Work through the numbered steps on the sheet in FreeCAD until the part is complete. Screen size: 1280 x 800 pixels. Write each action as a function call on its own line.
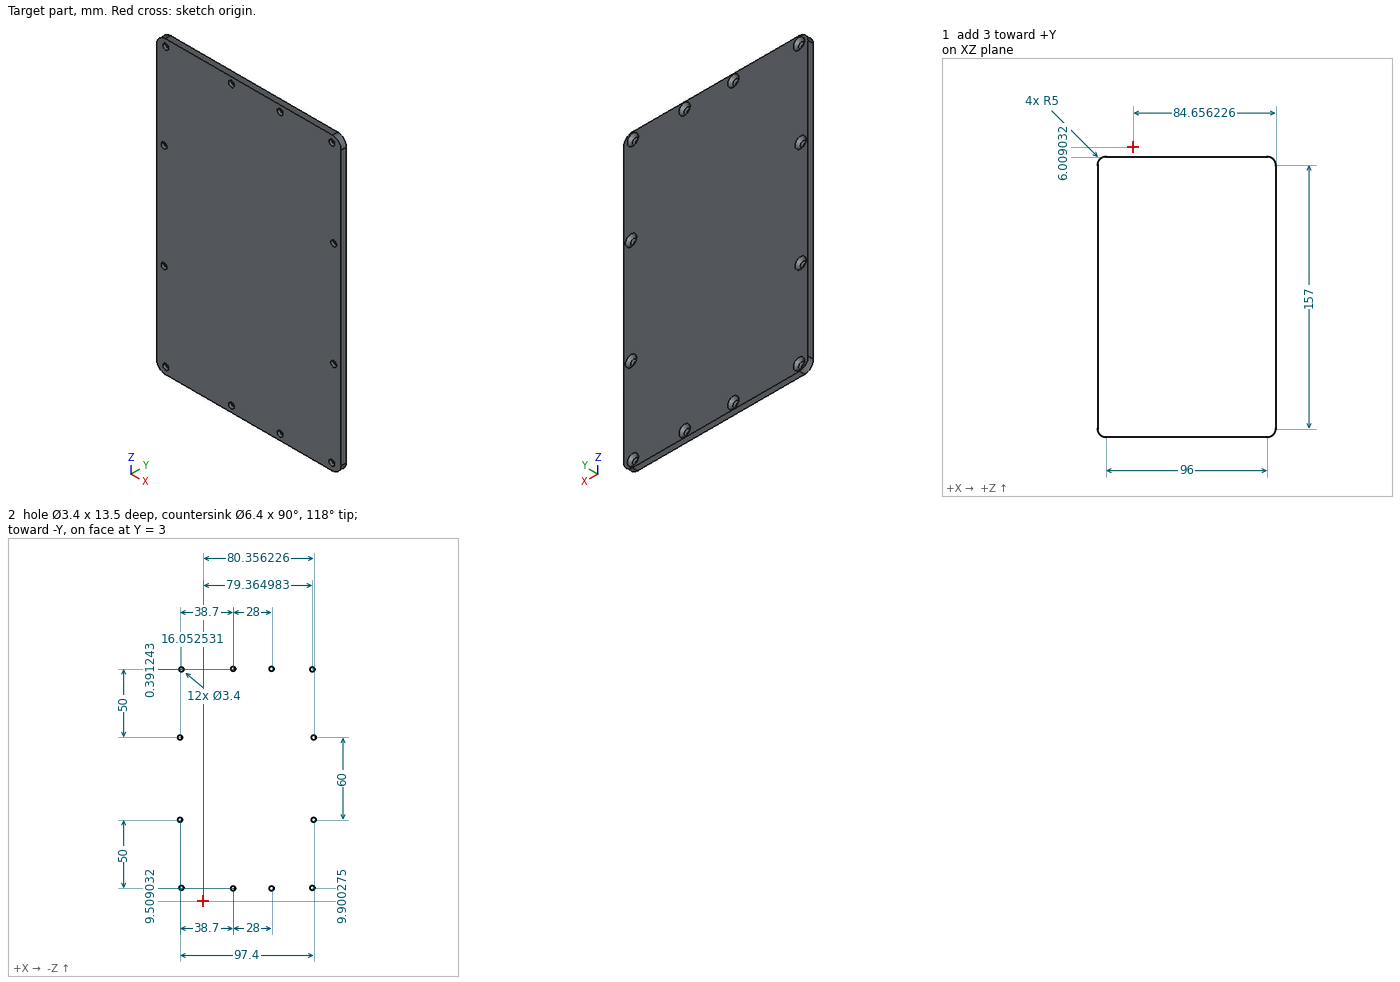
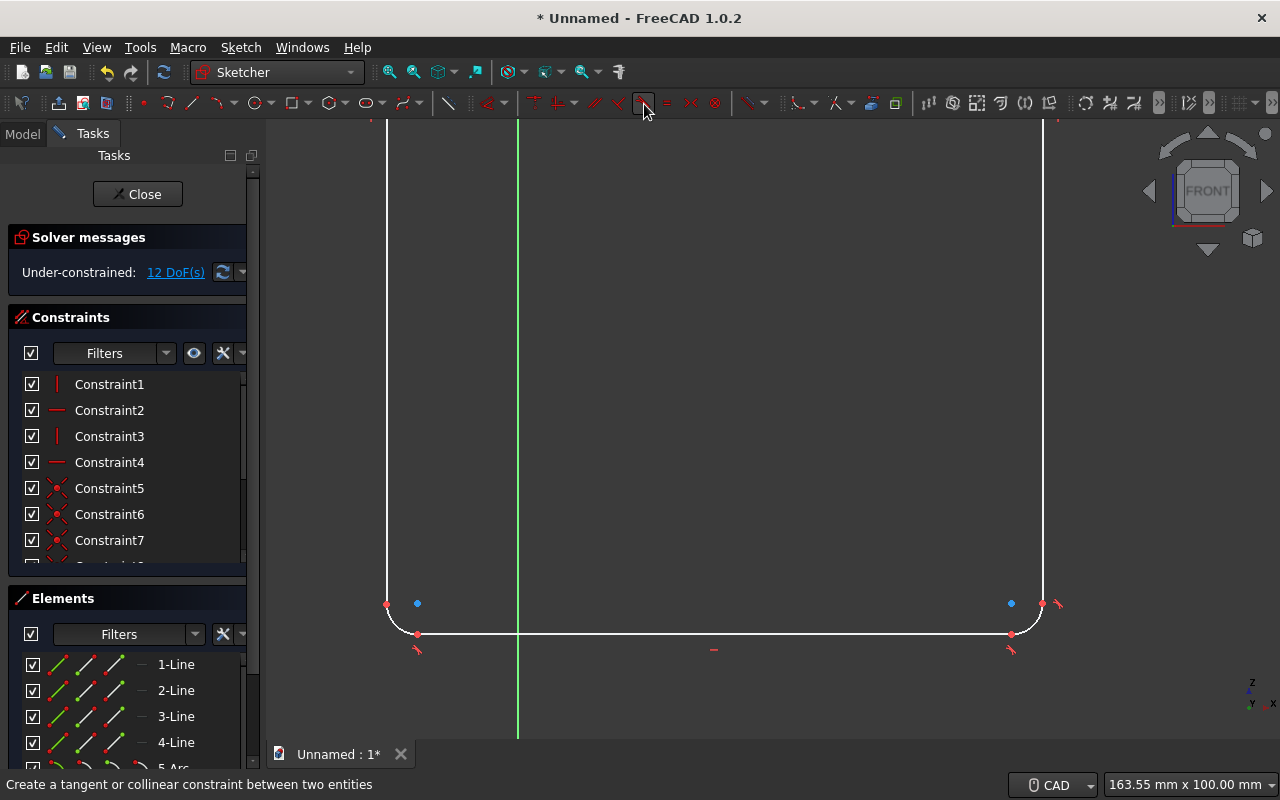
click(387, 313)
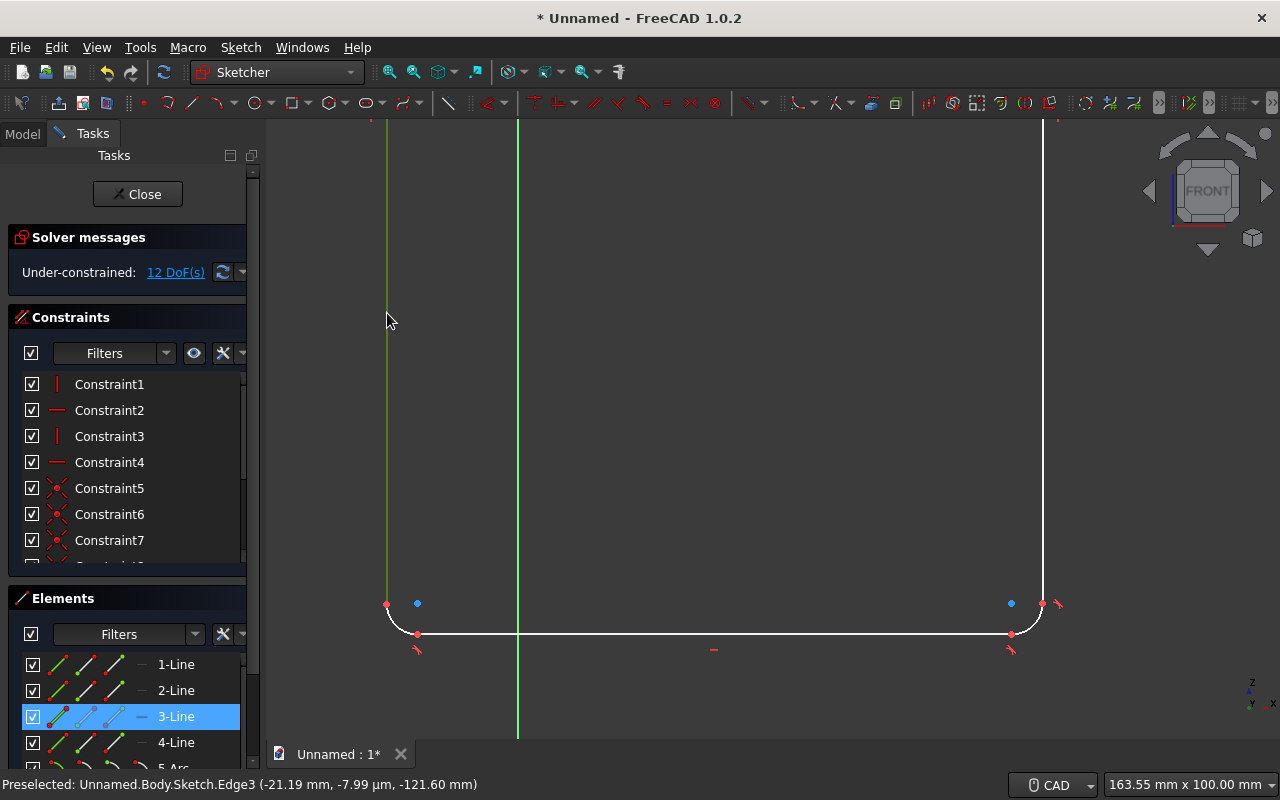
click(390, 618)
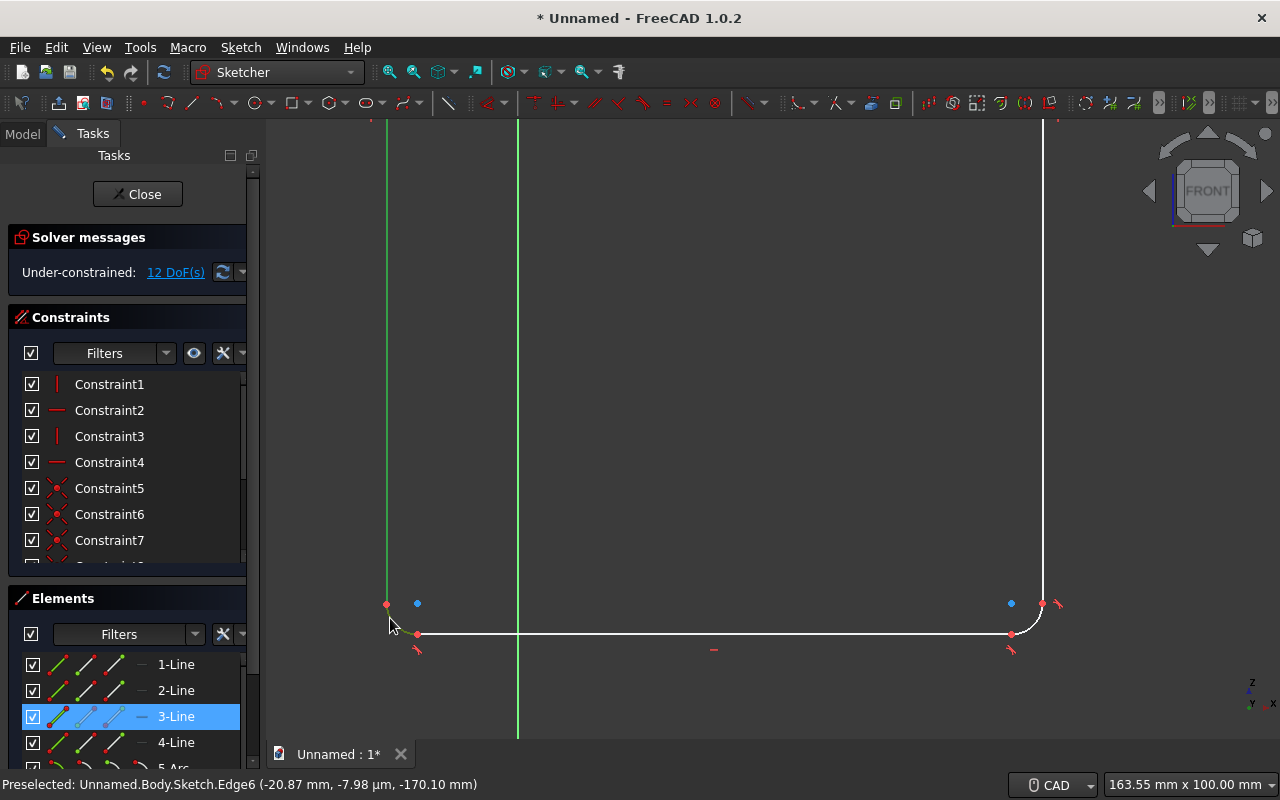
click(644, 104)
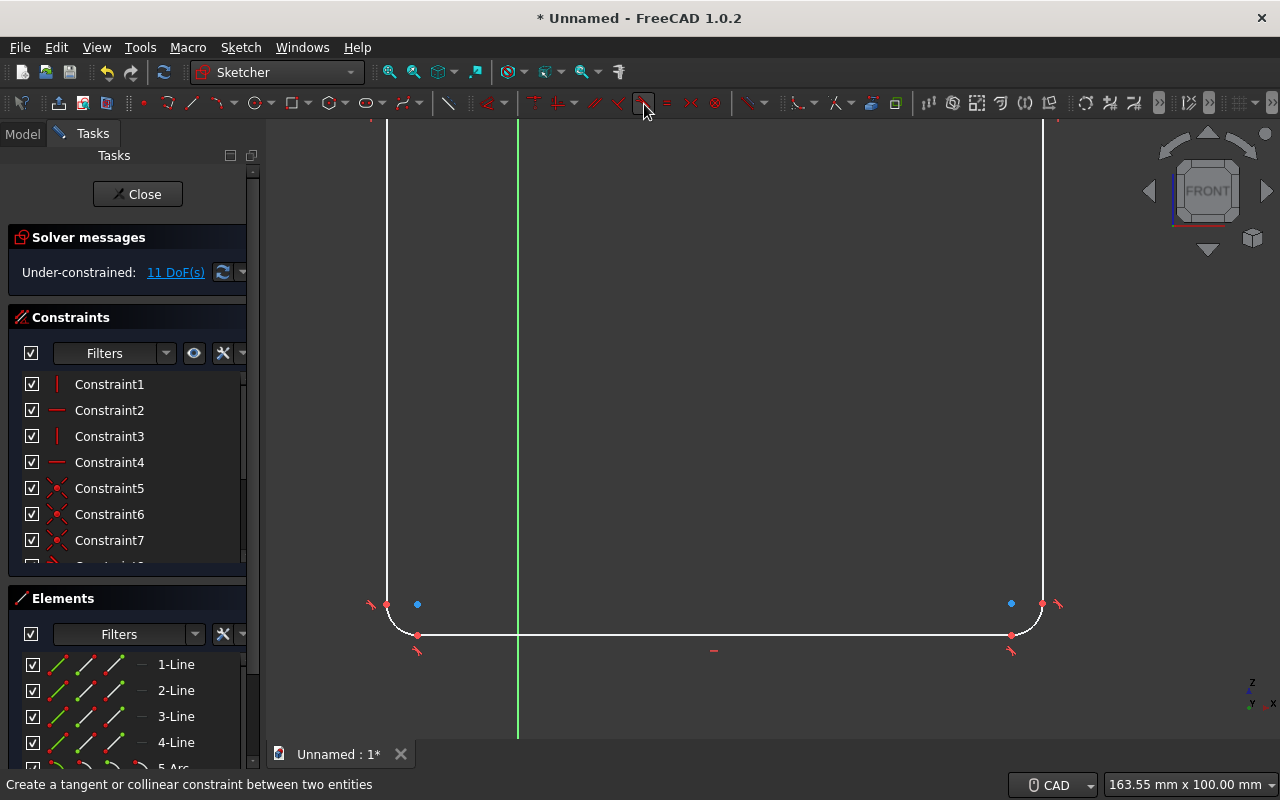
click(387, 313)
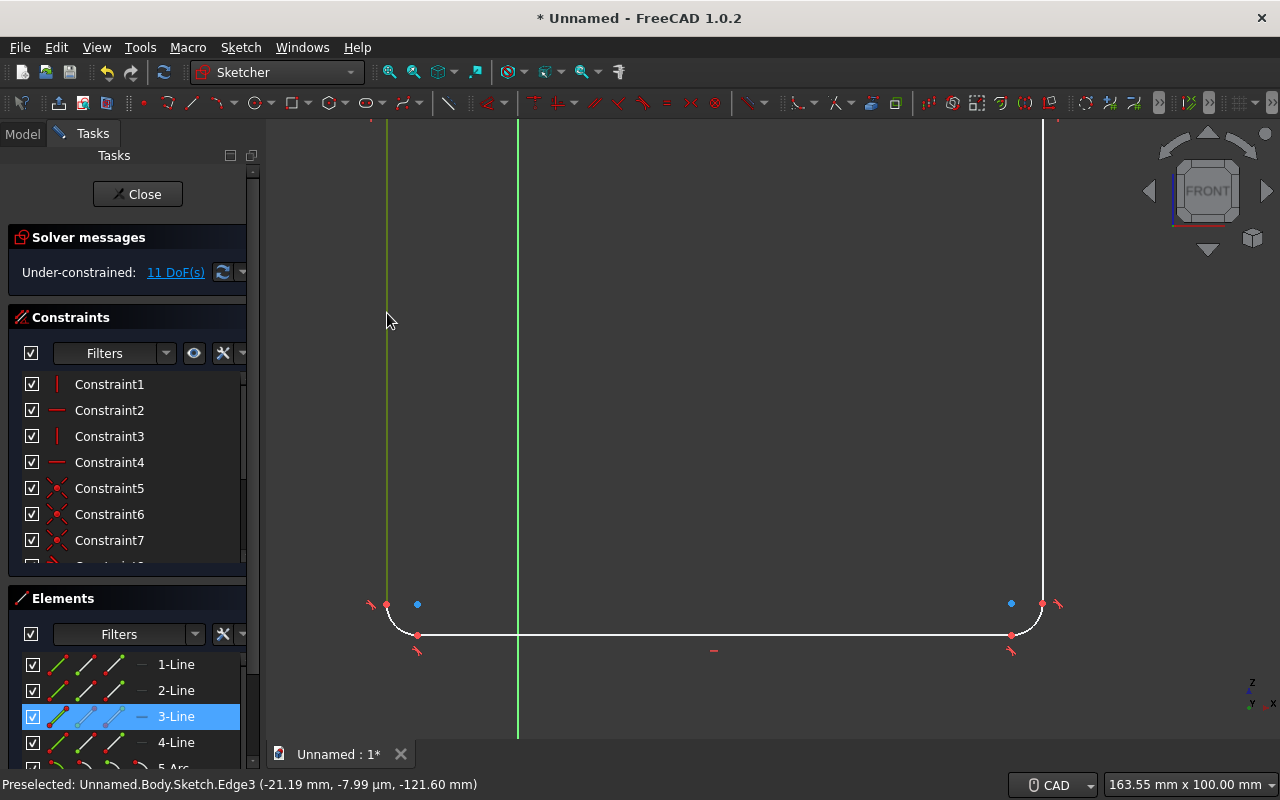
scroll(699, 623, down, 5)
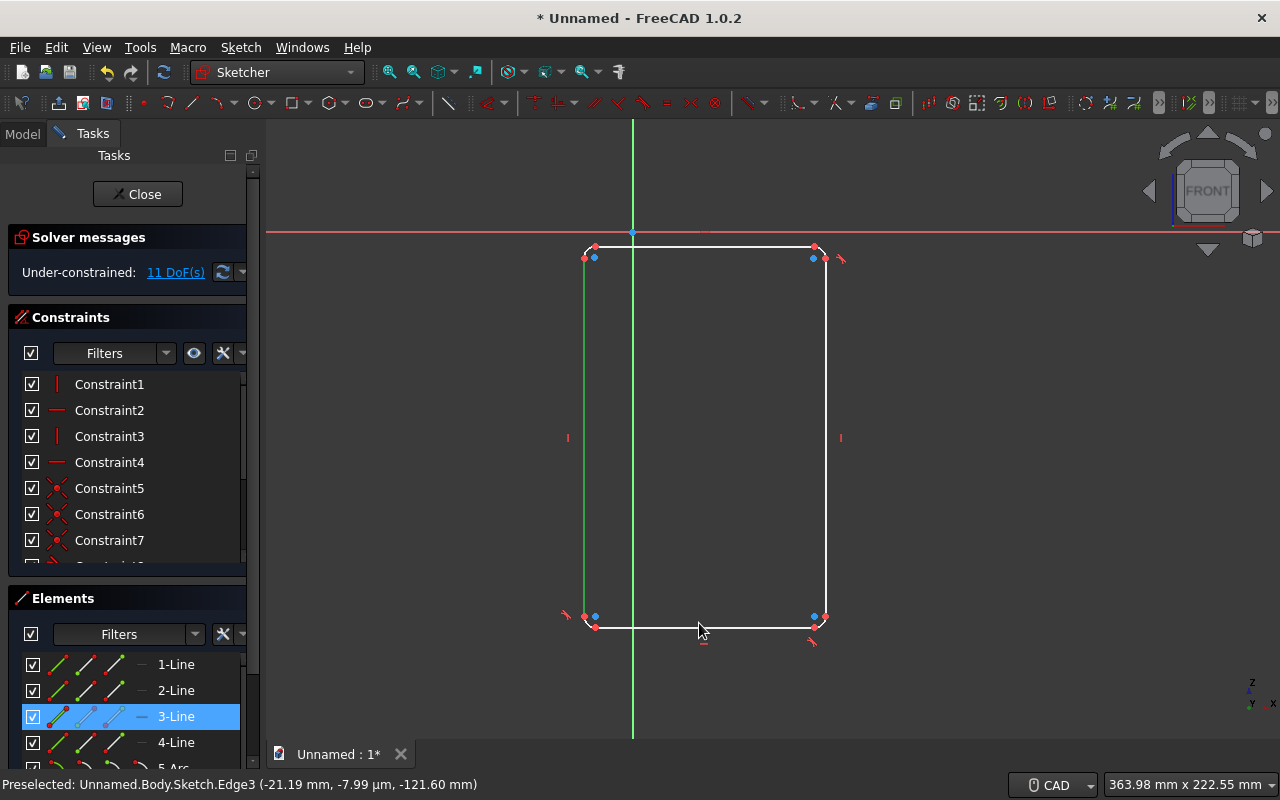
scroll(590, 248, up, 5)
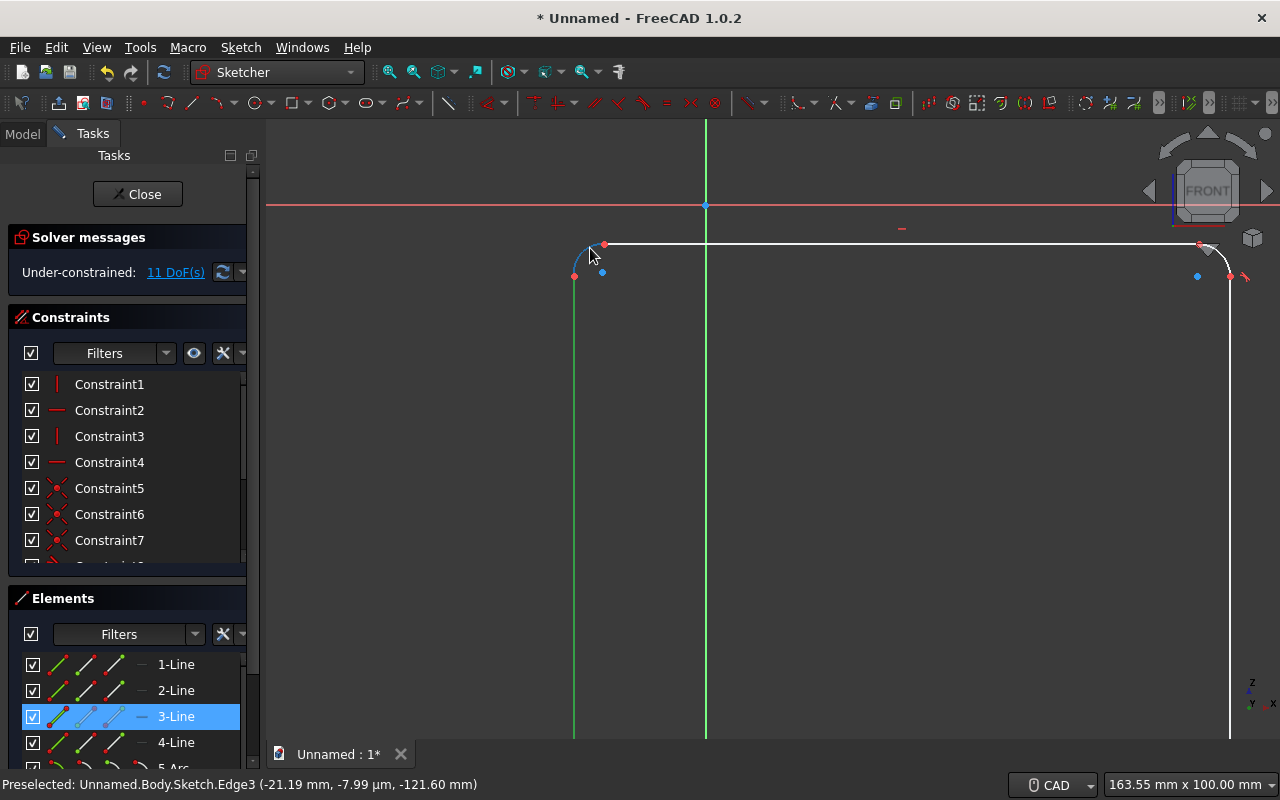
click(590, 247)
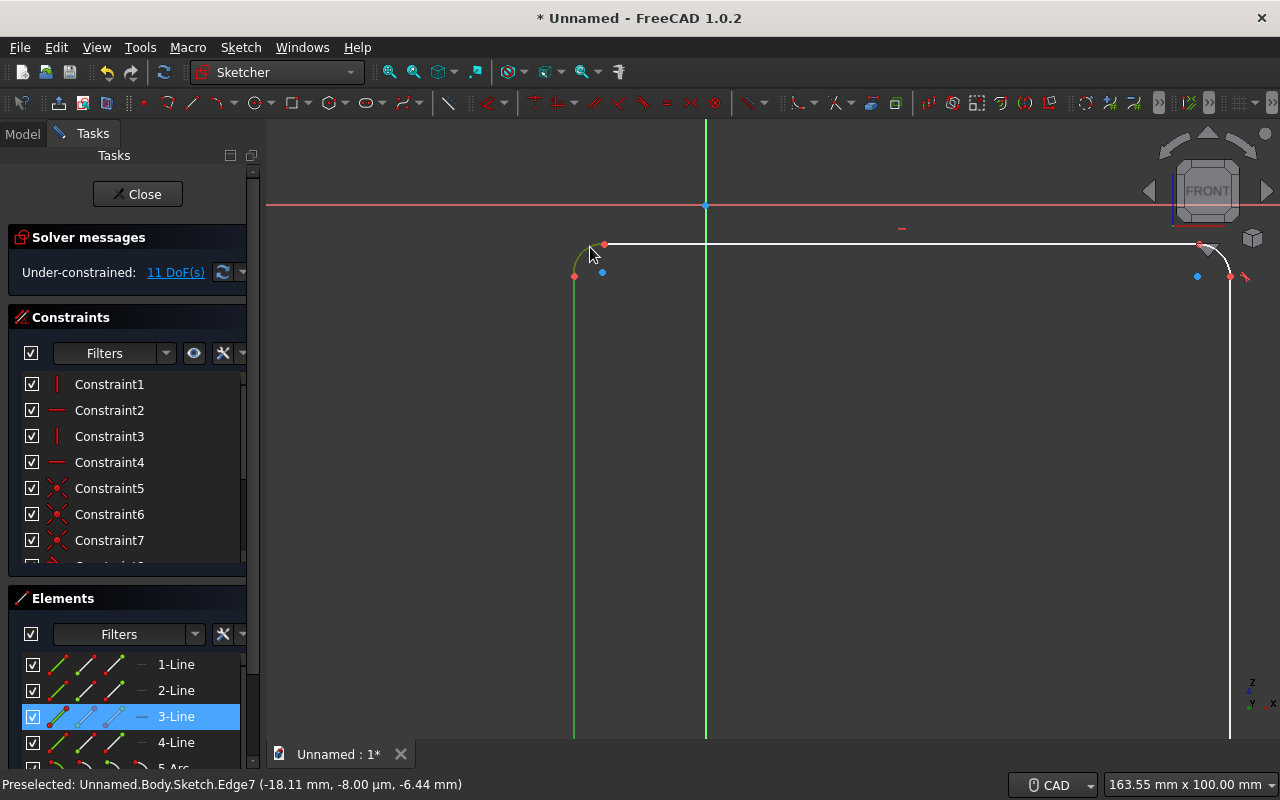
click(644, 104)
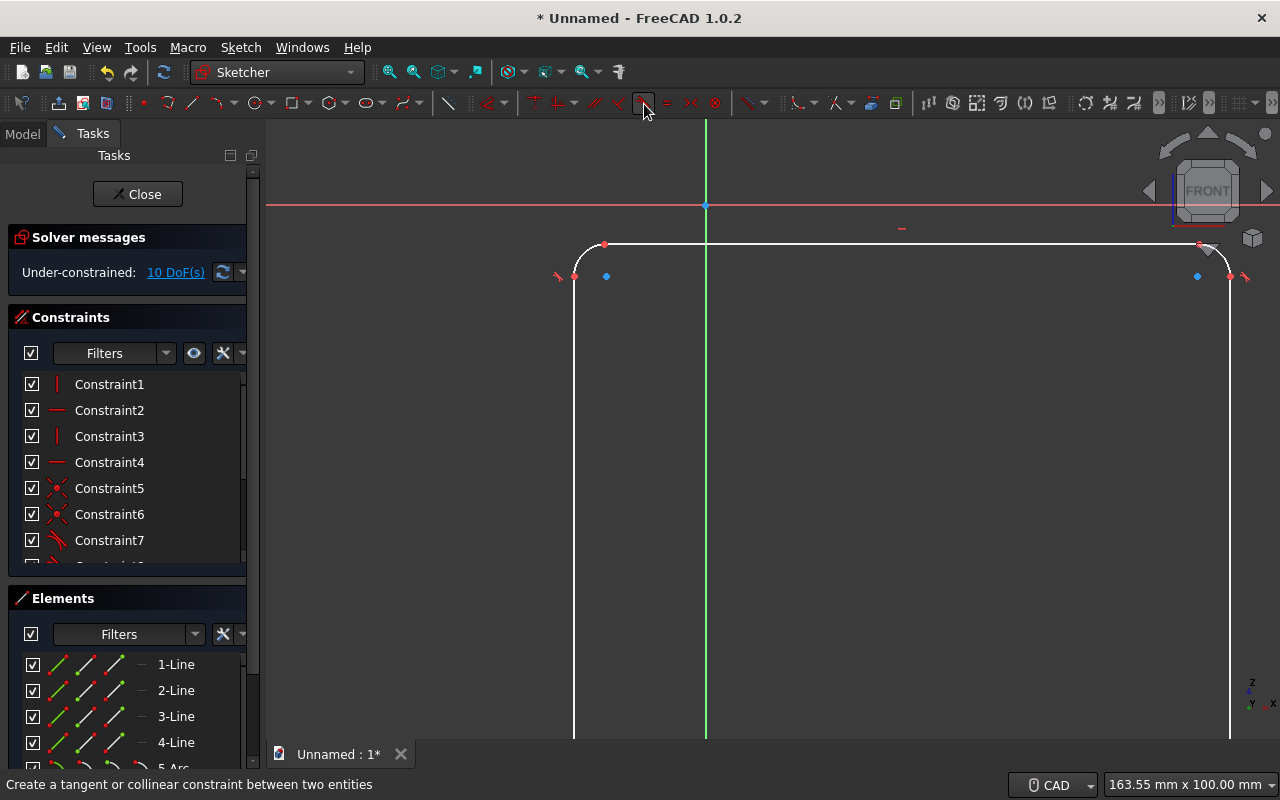
click(783, 244)